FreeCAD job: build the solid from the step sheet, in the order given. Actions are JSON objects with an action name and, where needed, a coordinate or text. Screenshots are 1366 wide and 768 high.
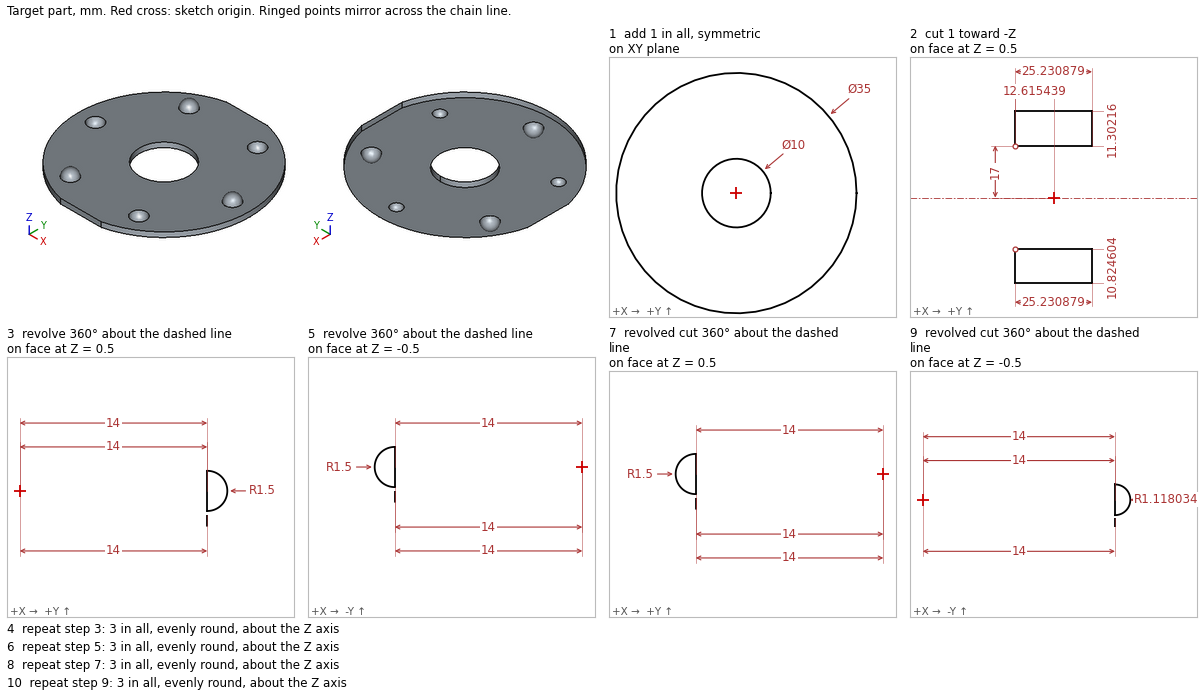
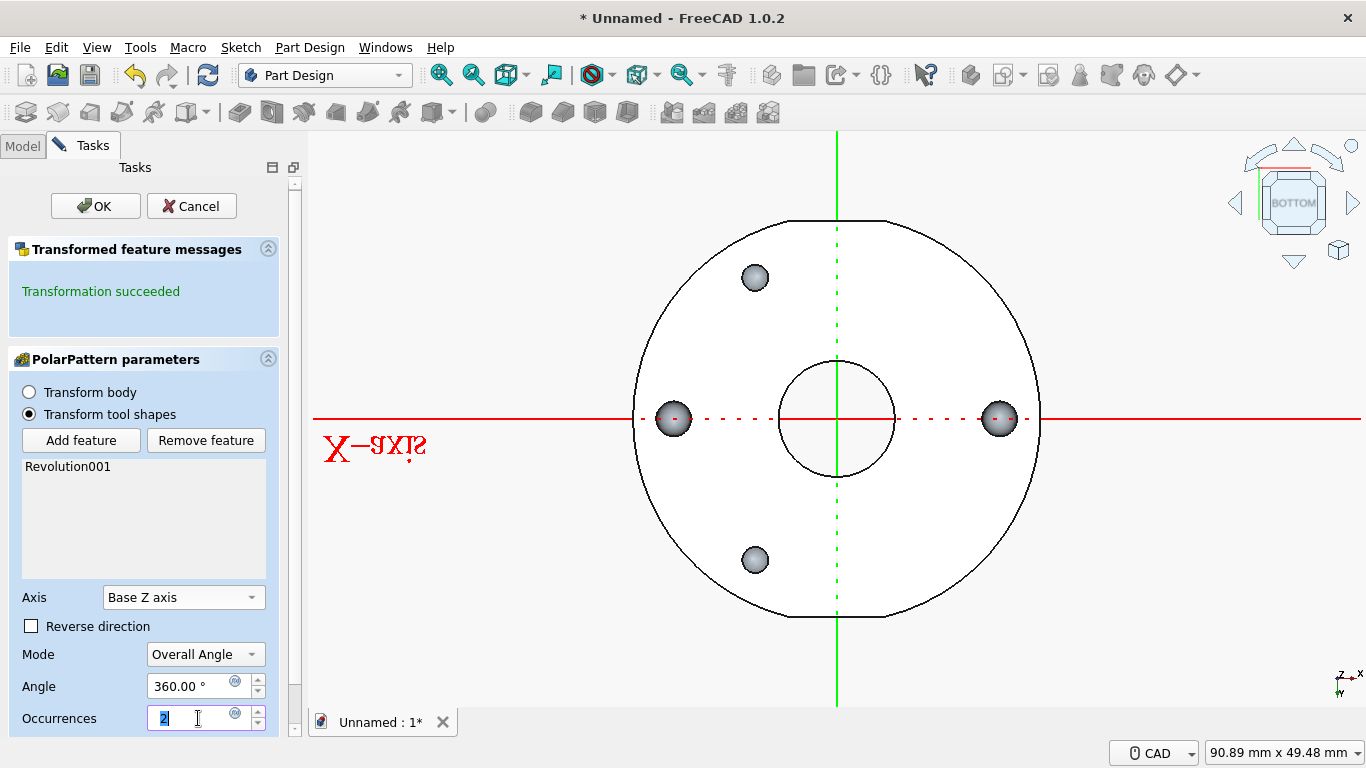
{"action": "type", "text": "3"}
{"action": "key", "text": "Tab"}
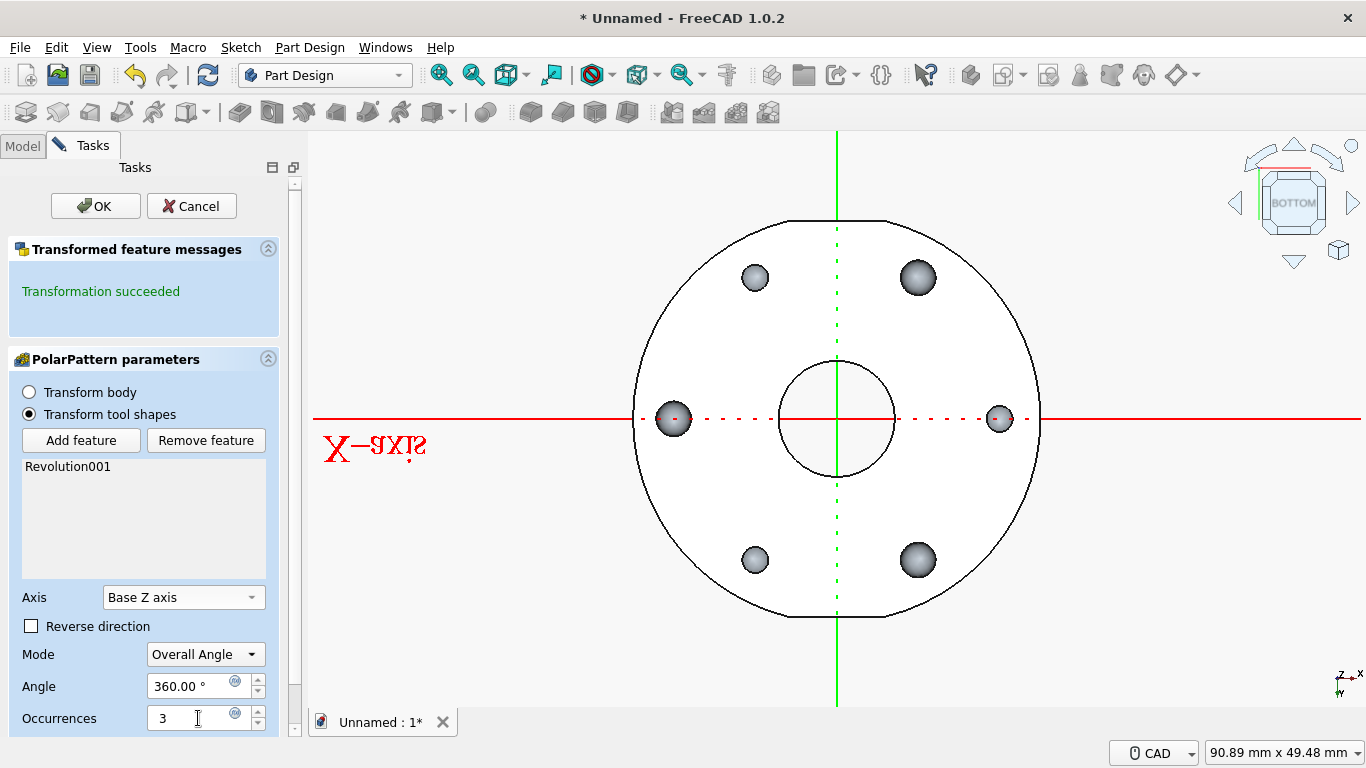
{"action": "left_click", "coordinate": [96, 206]}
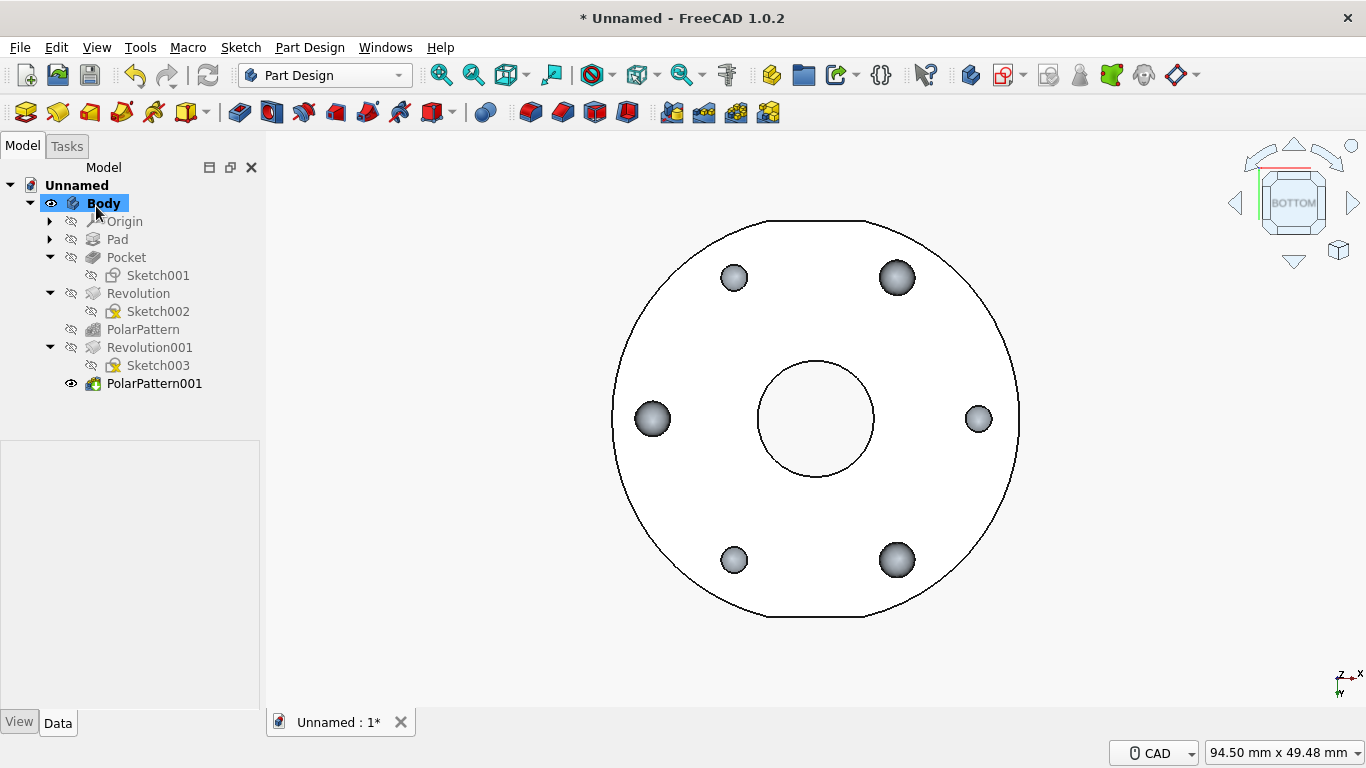
{"action": "key", "text": "0"}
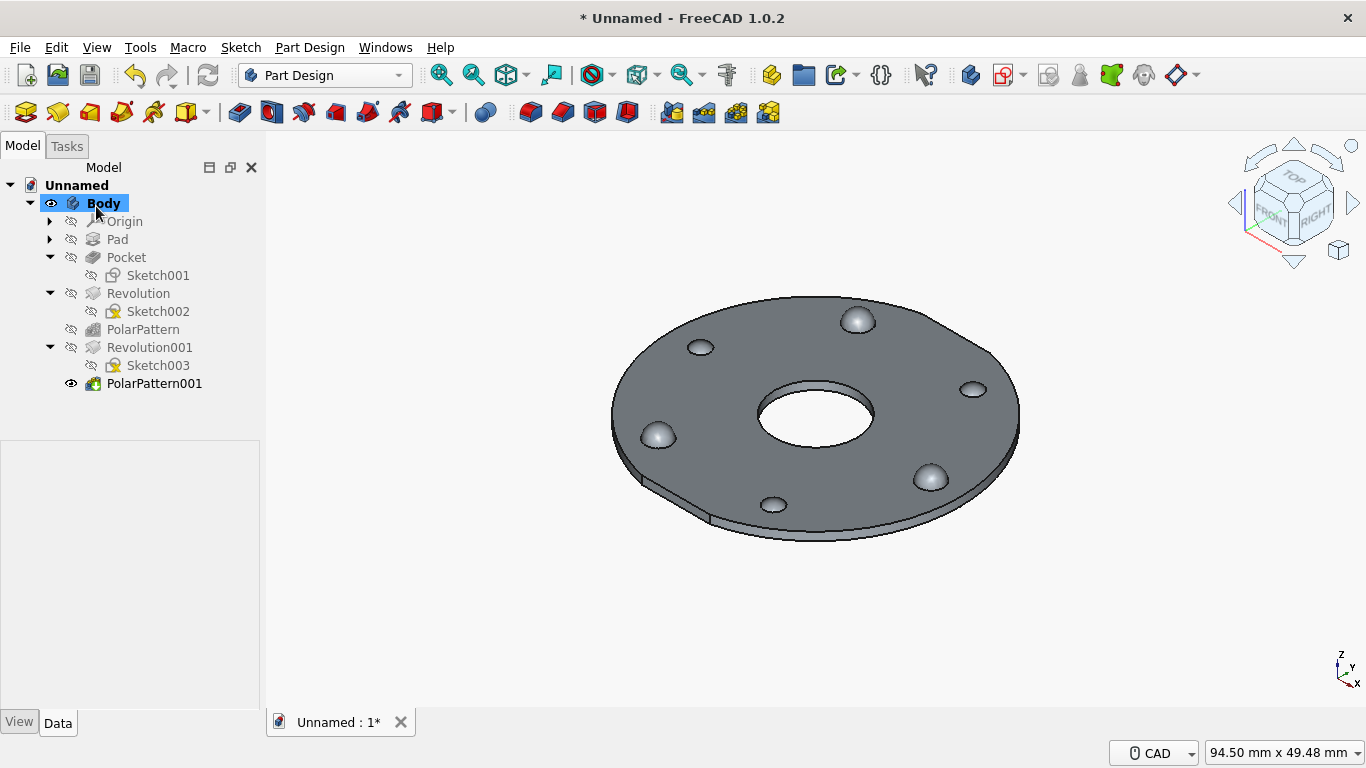
{"action": "left_click", "coordinate": [693, 389]}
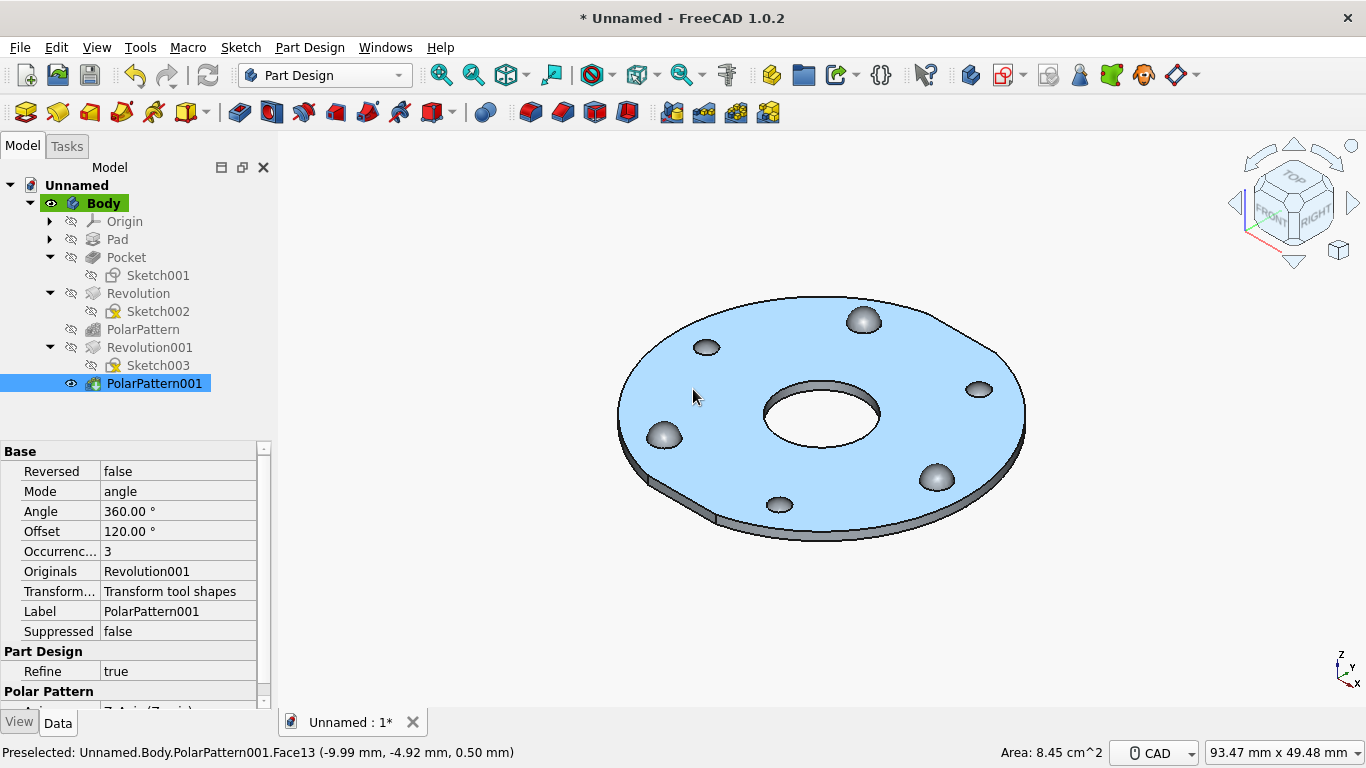
{"action": "left_click", "coordinate": [1004, 76]}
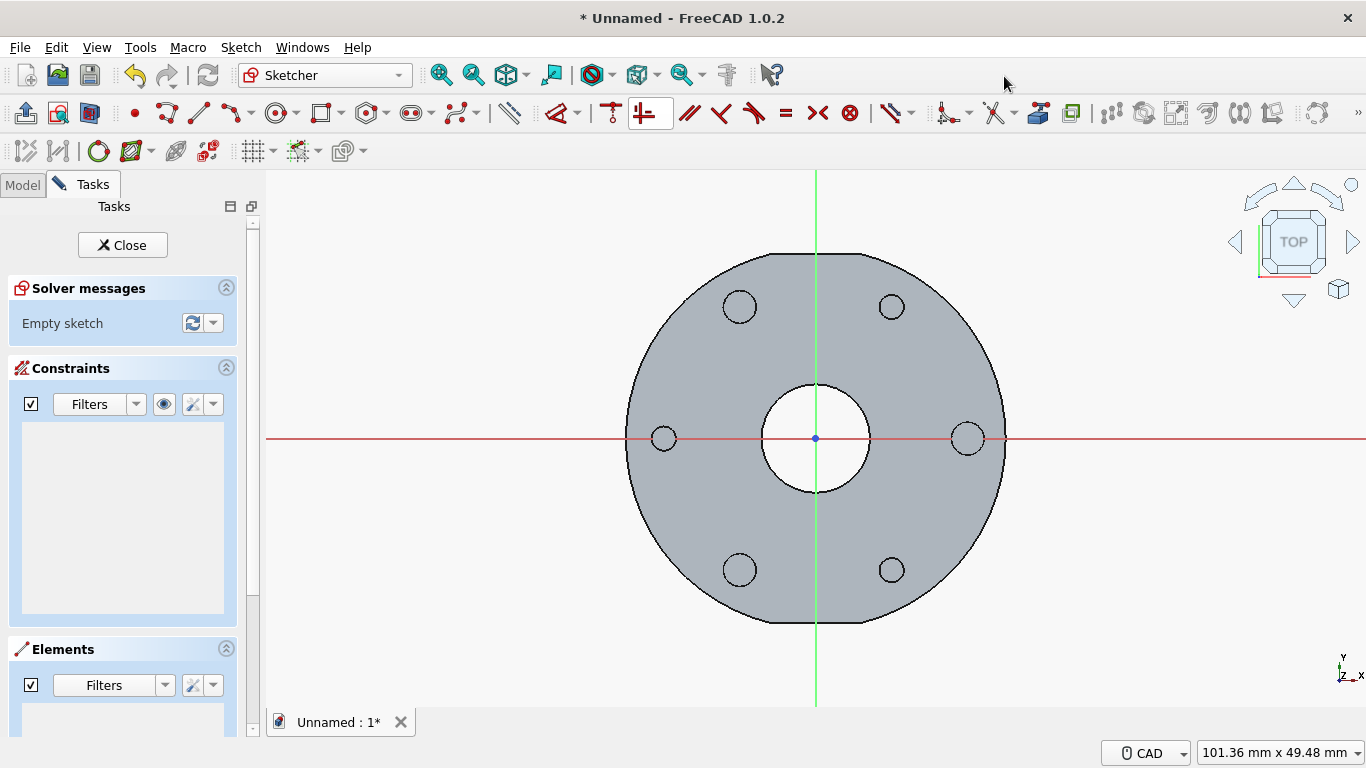
{"action": "scroll", "coordinate": [641, 446], "scroll_direction": "up", "scroll_amount": 10}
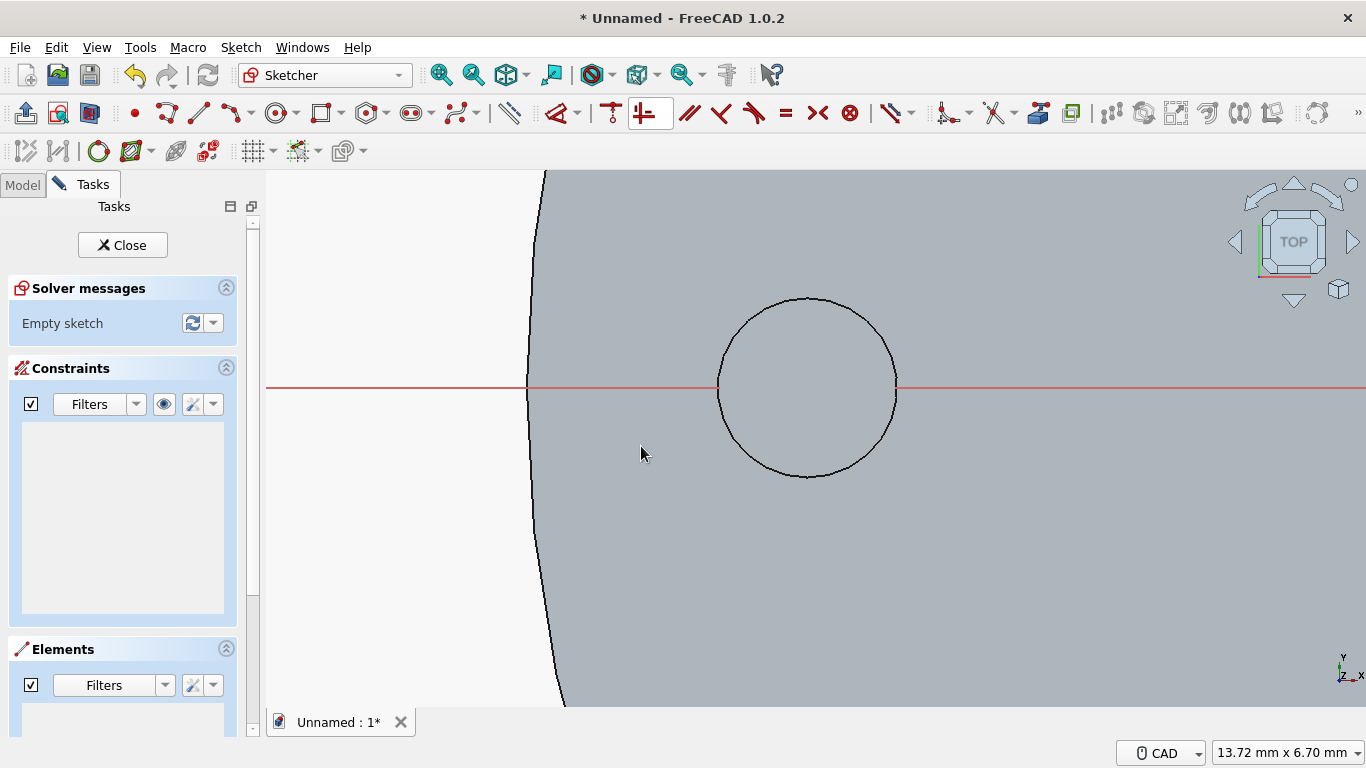
{"action": "key", "text": "g l"}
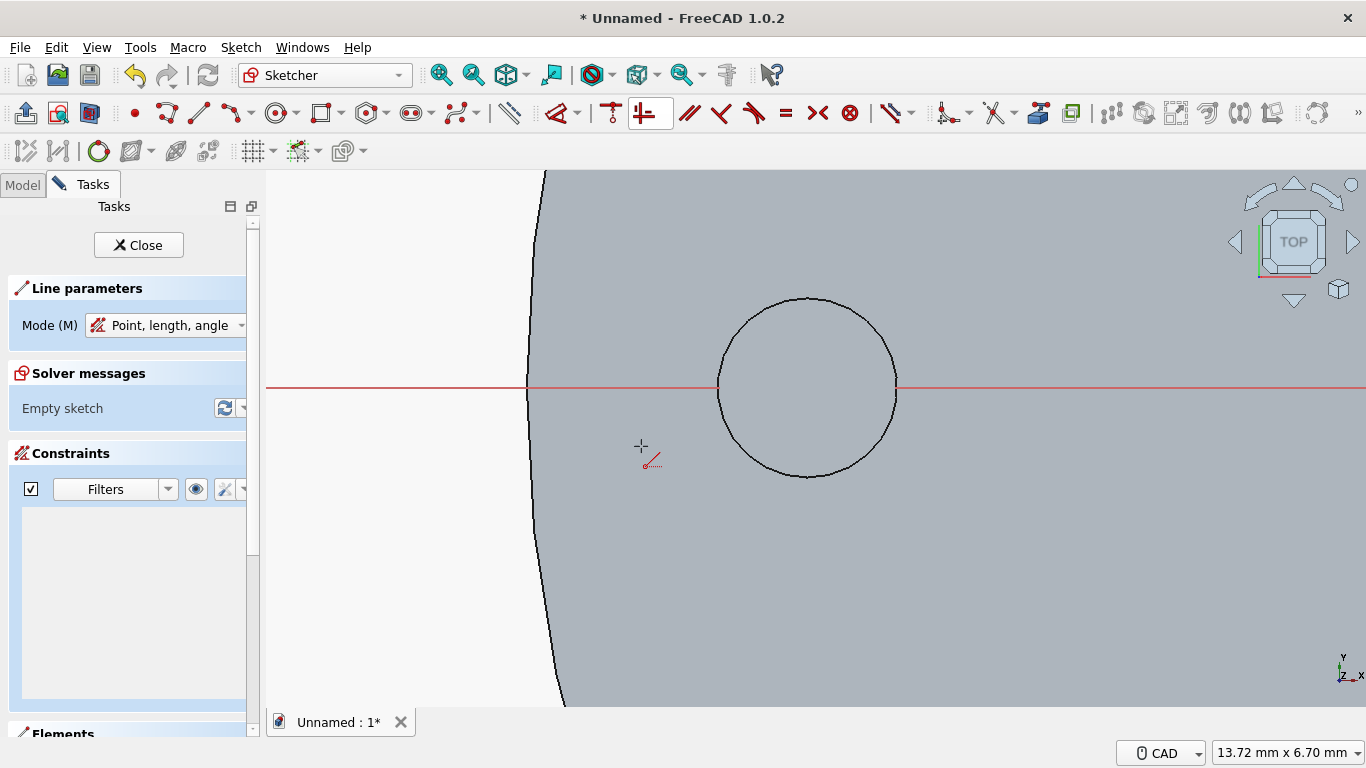
{"action": "left_click", "coordinate": [807, 508]}
{"action": "left_click", "coordinate": [807, 268]}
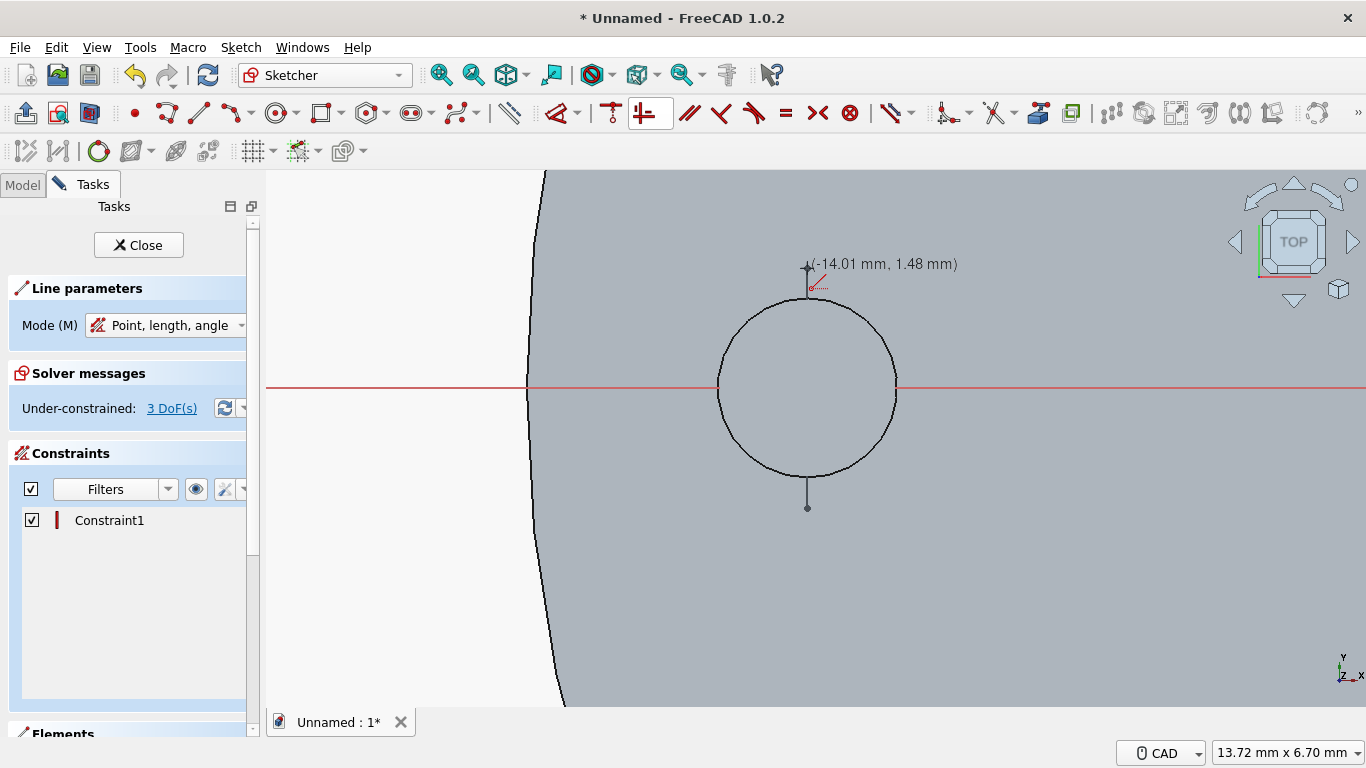
{"action": "key", "text": "g 3 a"}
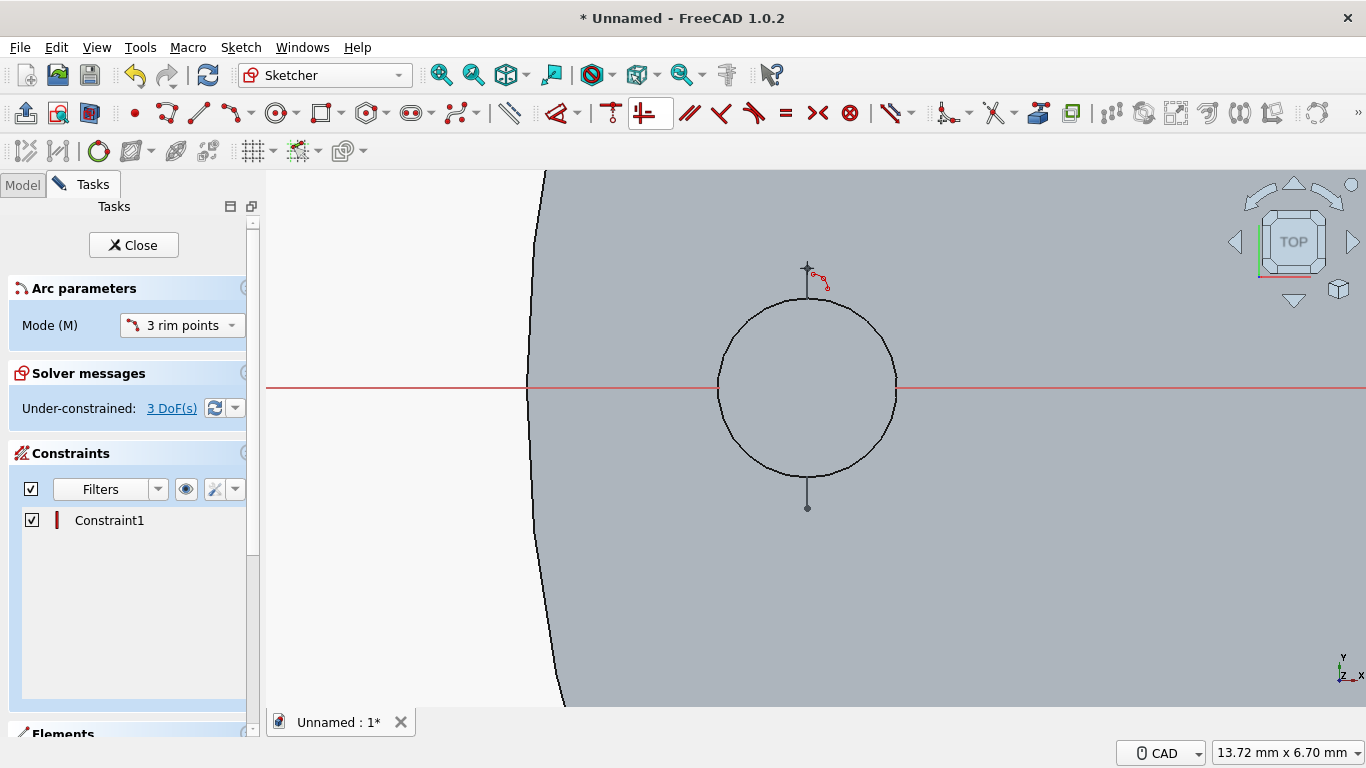
{"action": "left_click", "coordinate": [807, 269]}
{"action": "left_click", "coordinate": [807, 509]}
{"action": "left_click", "coordinate": [693, 351]}